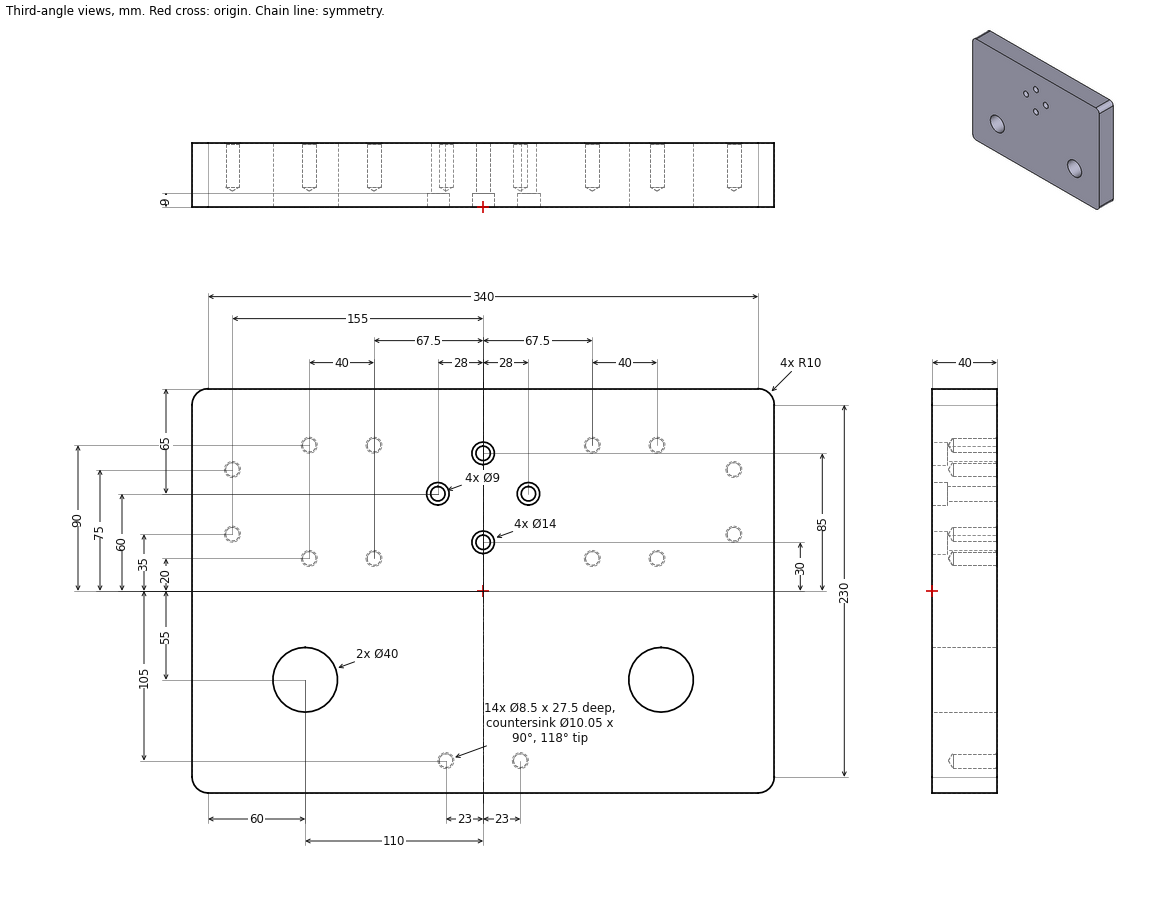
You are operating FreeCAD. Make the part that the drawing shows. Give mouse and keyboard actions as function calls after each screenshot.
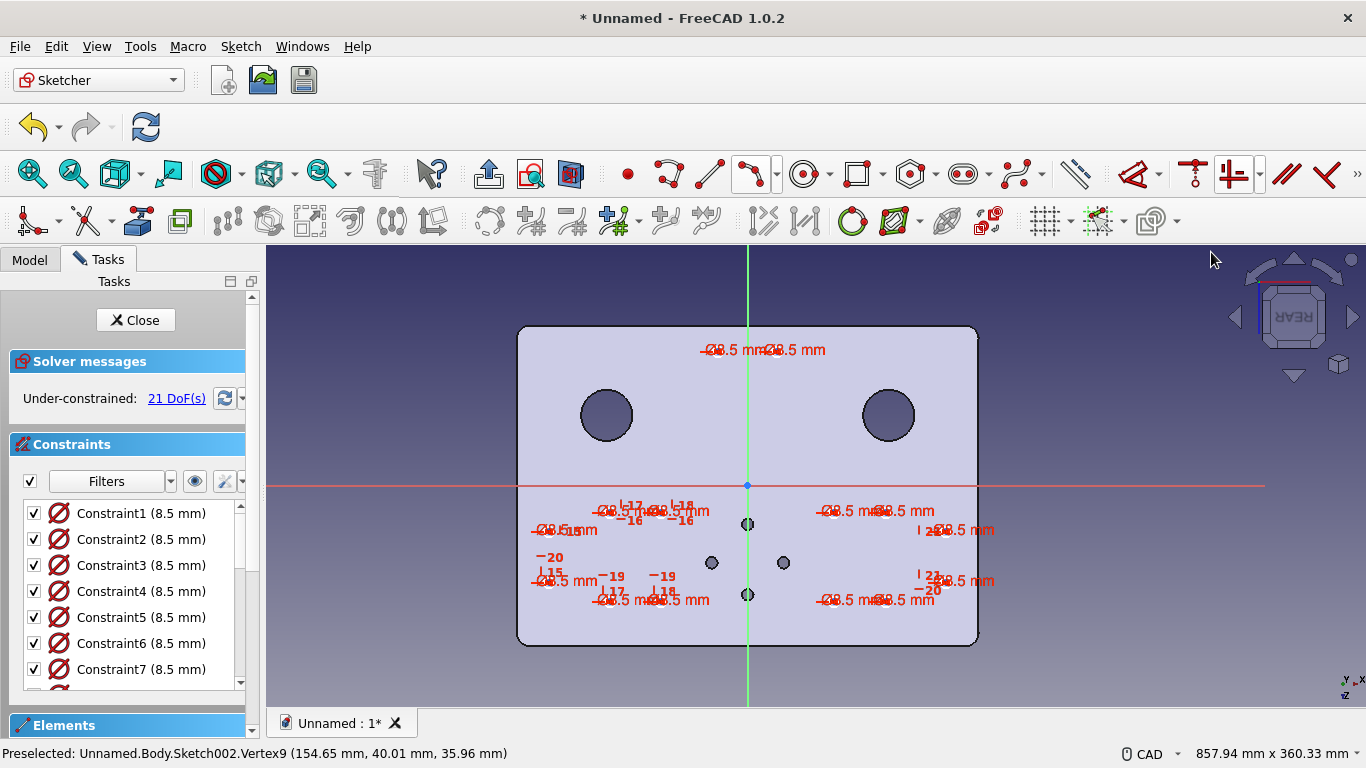
click(661, 602)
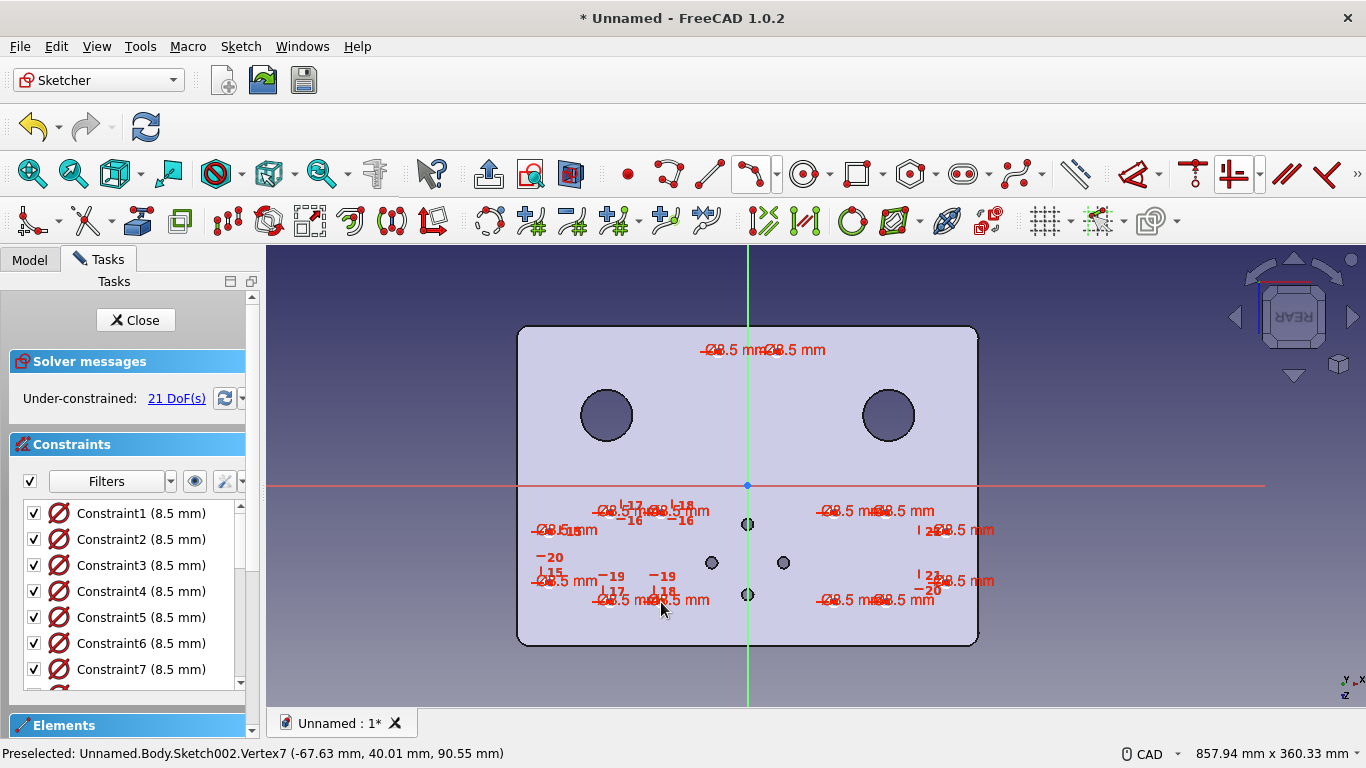
click(834, 602)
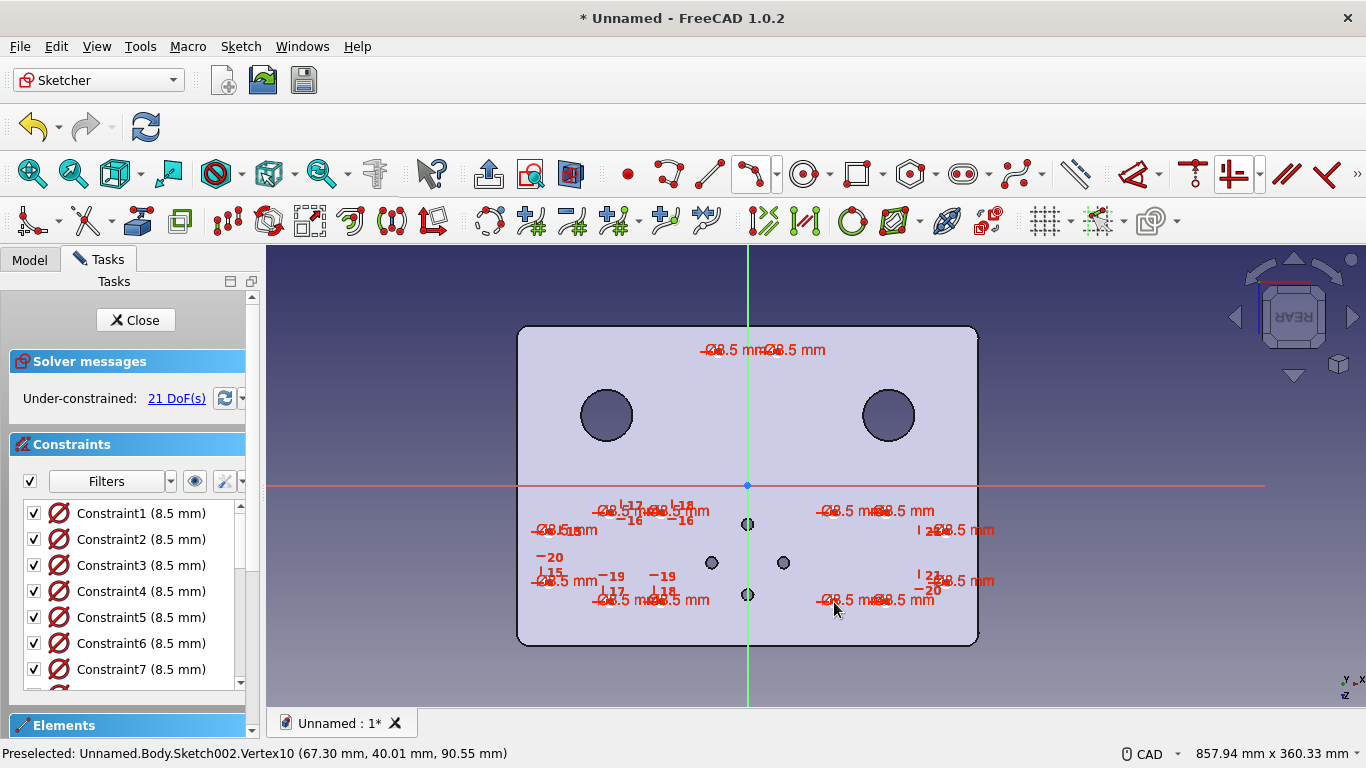
click(1260, 174)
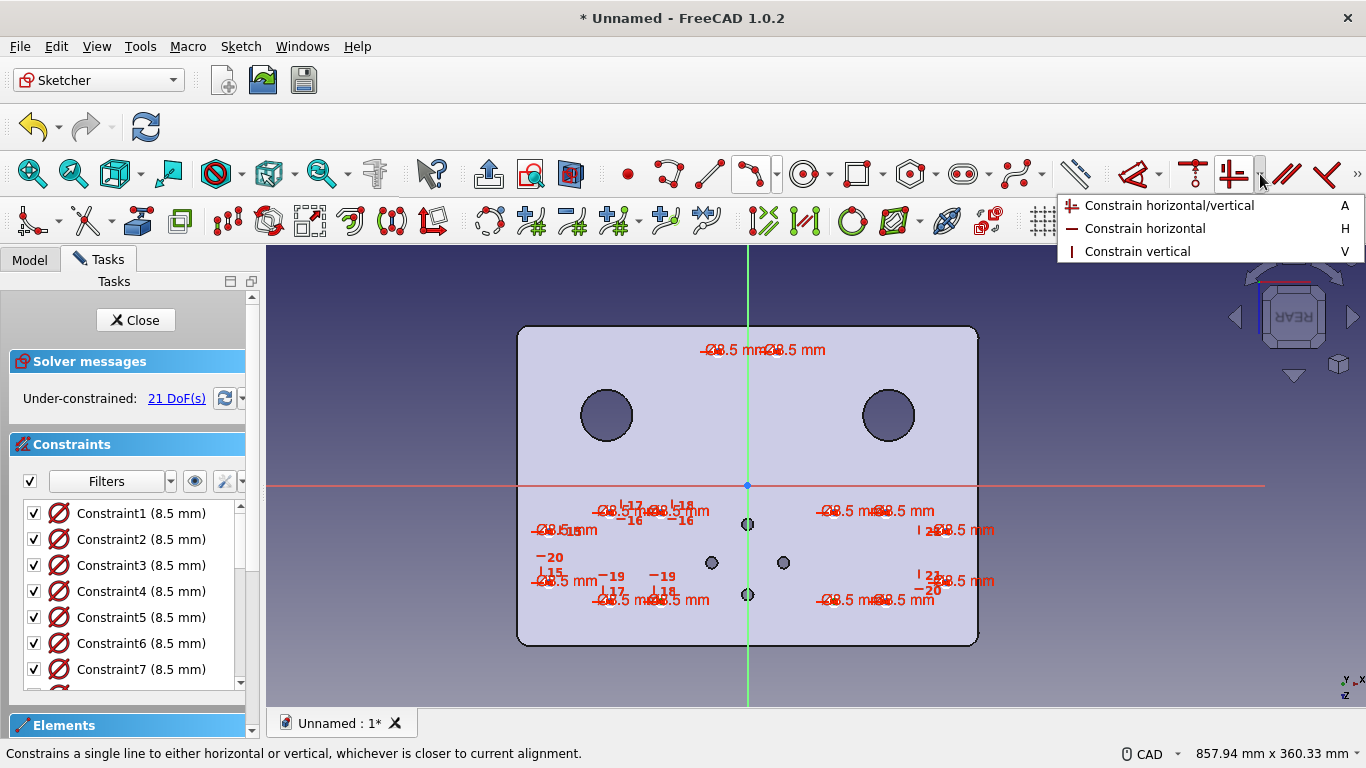
click(1211, 228)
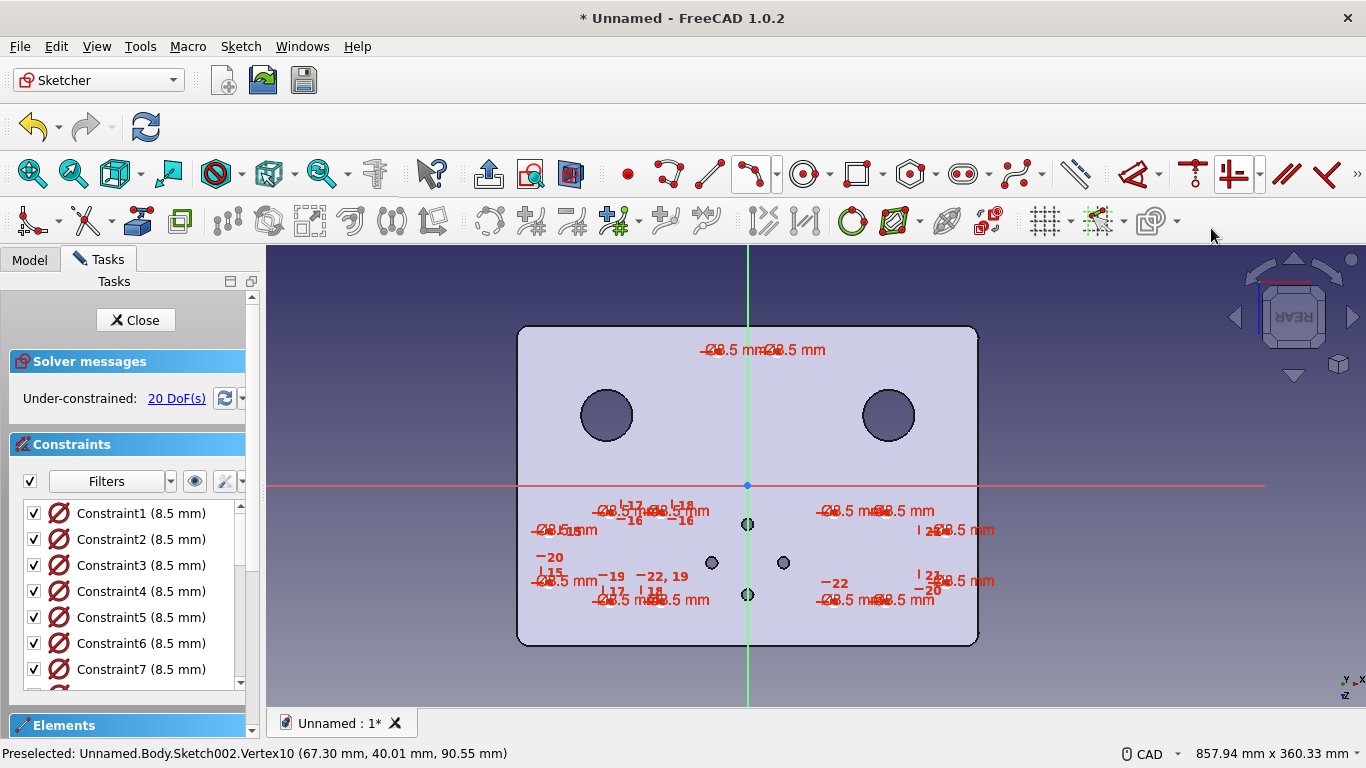
click(834, 602)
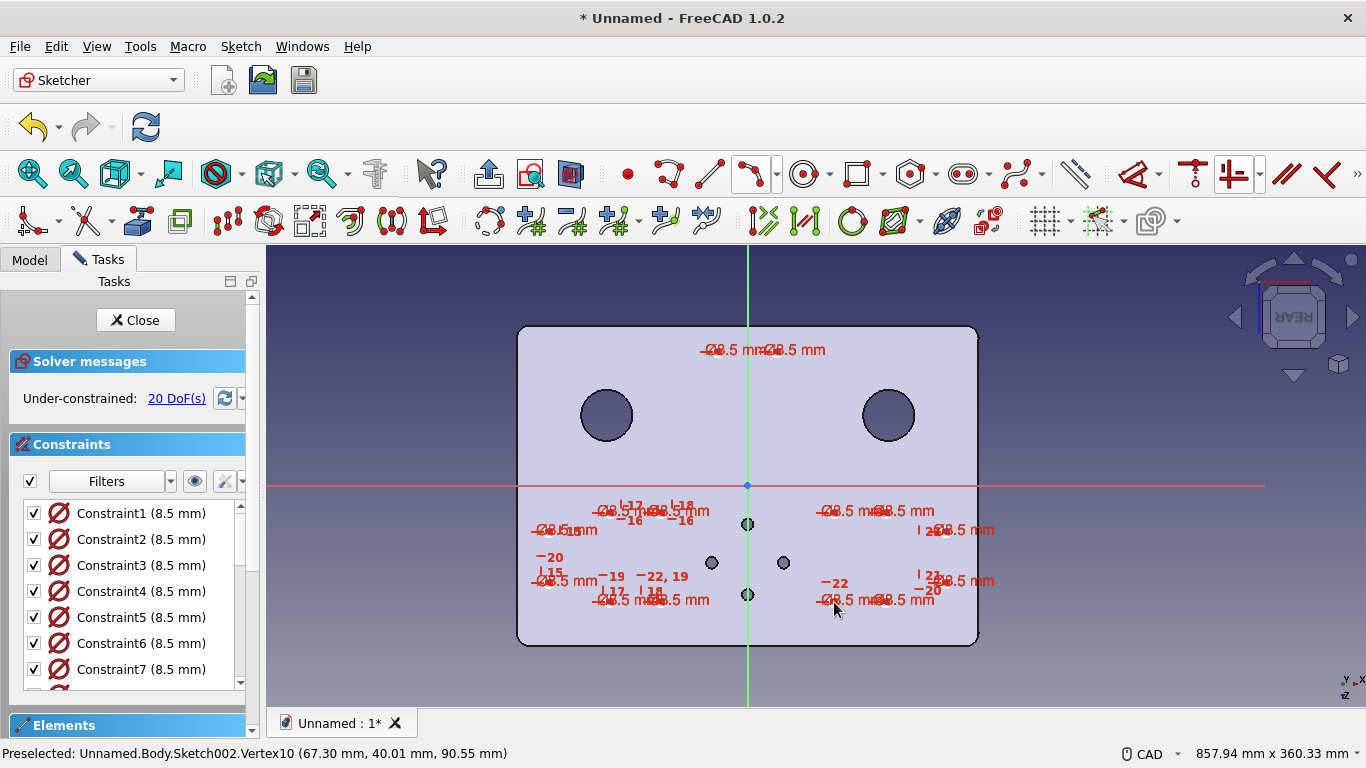
click(886, 602)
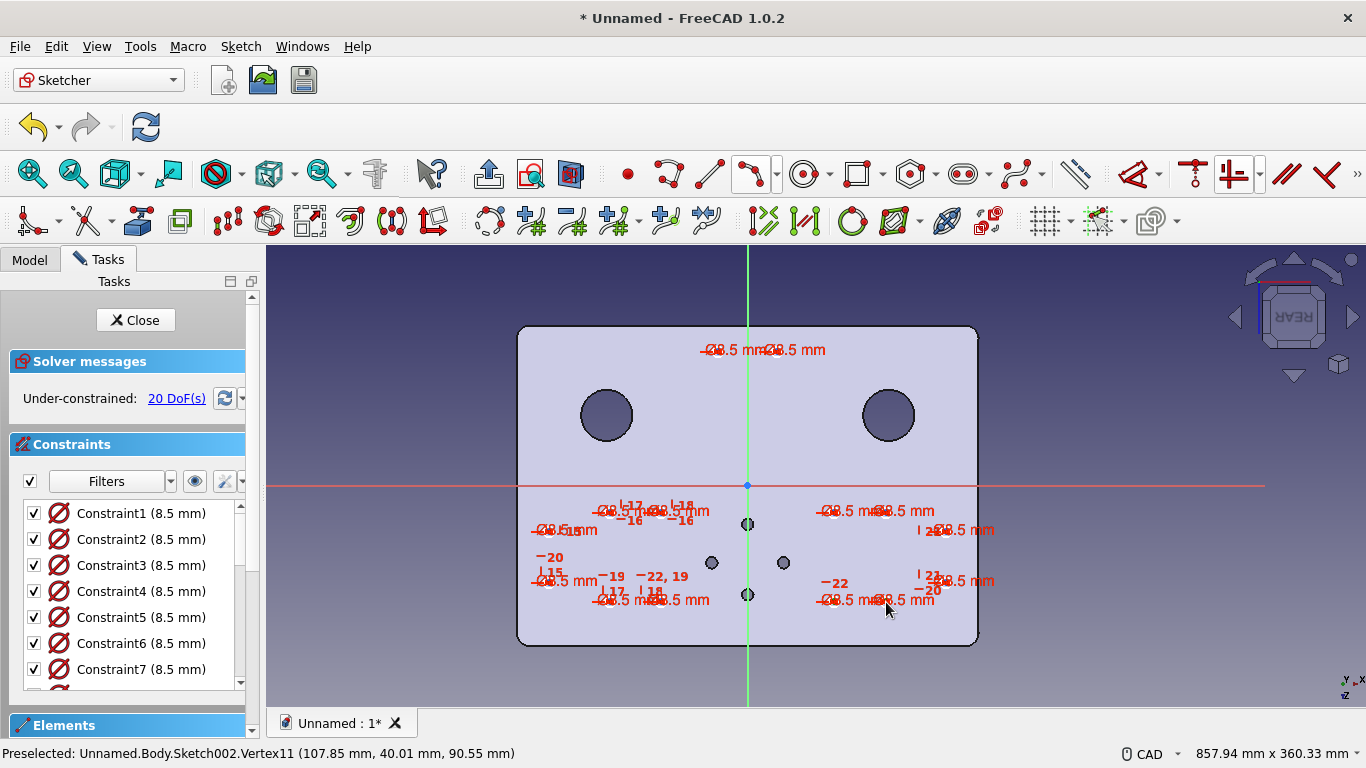
key(h)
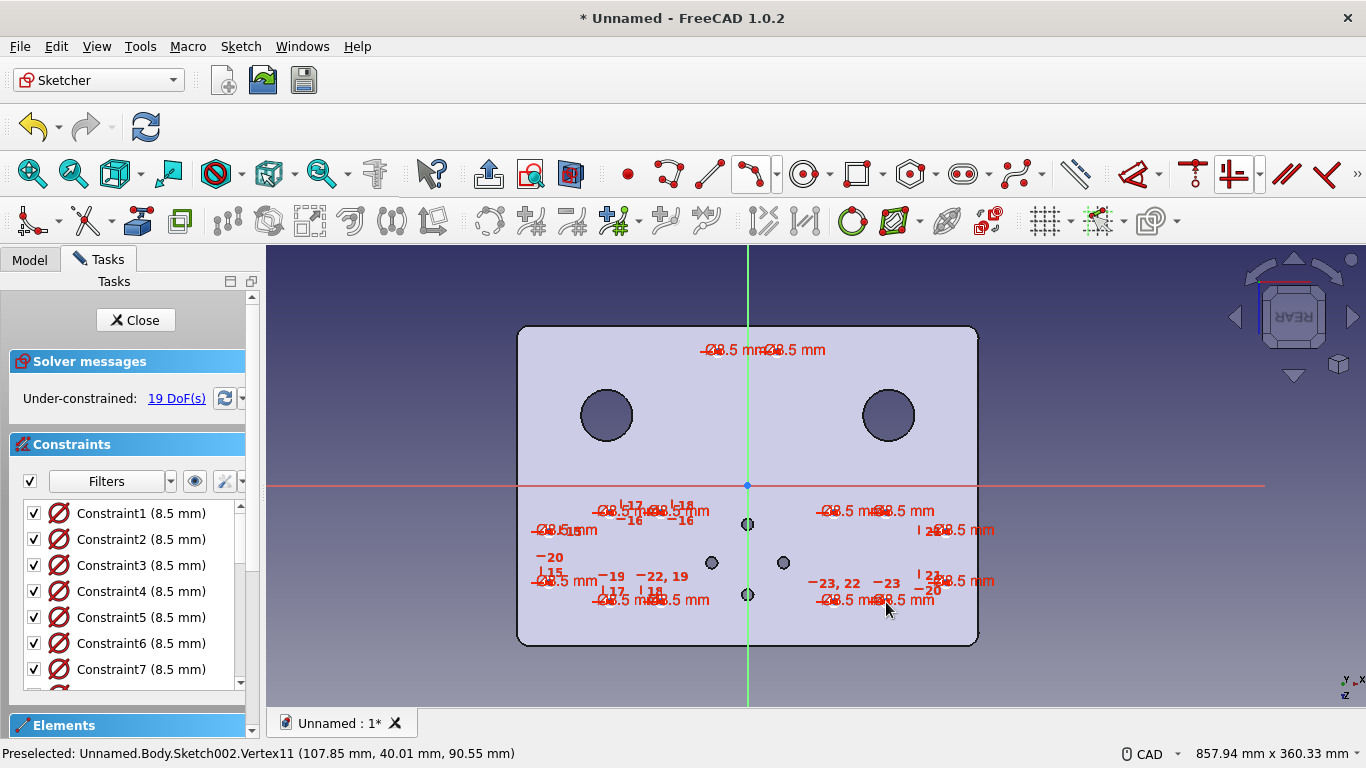
click(834, 602)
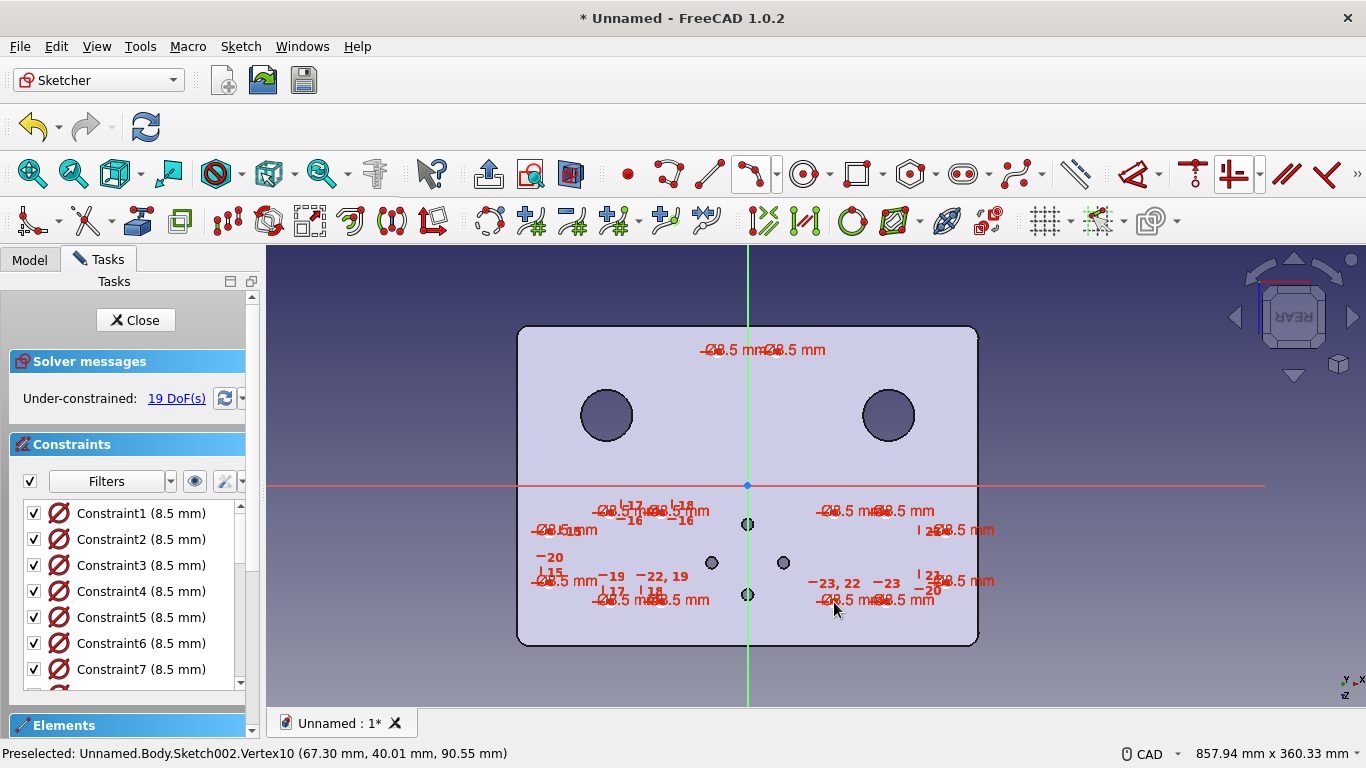
click(834, 513)